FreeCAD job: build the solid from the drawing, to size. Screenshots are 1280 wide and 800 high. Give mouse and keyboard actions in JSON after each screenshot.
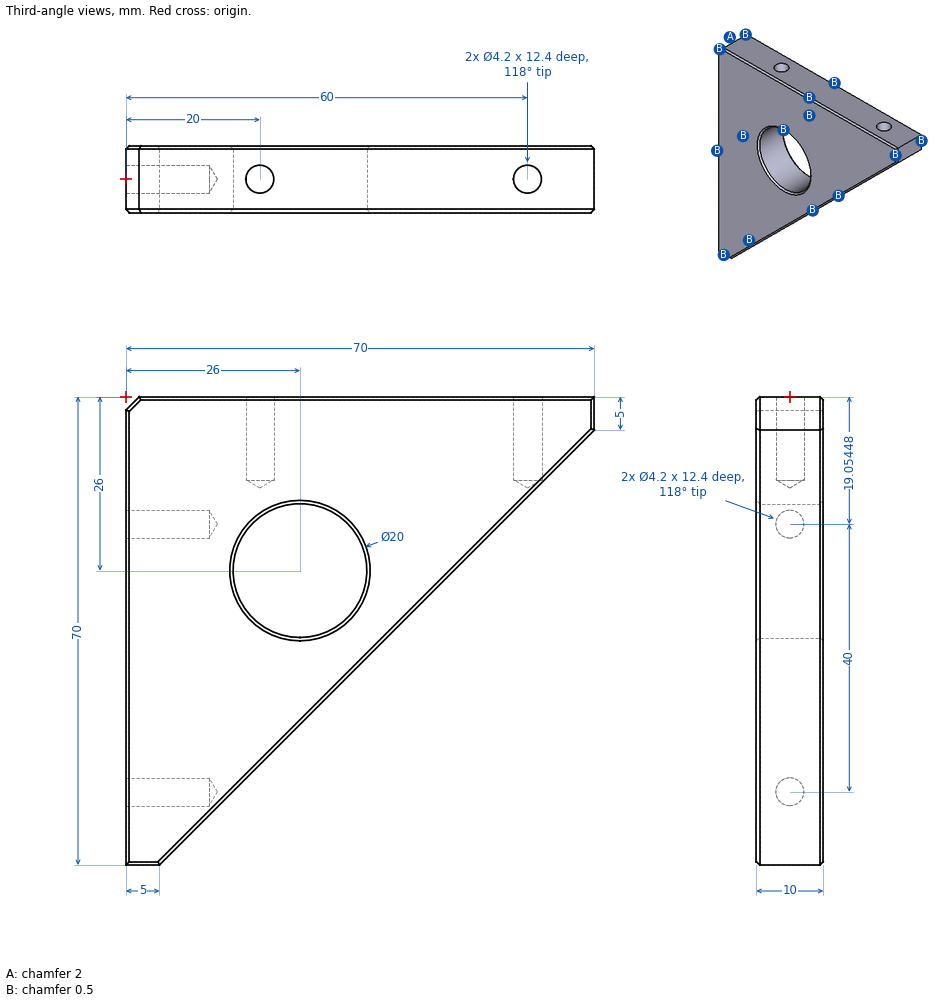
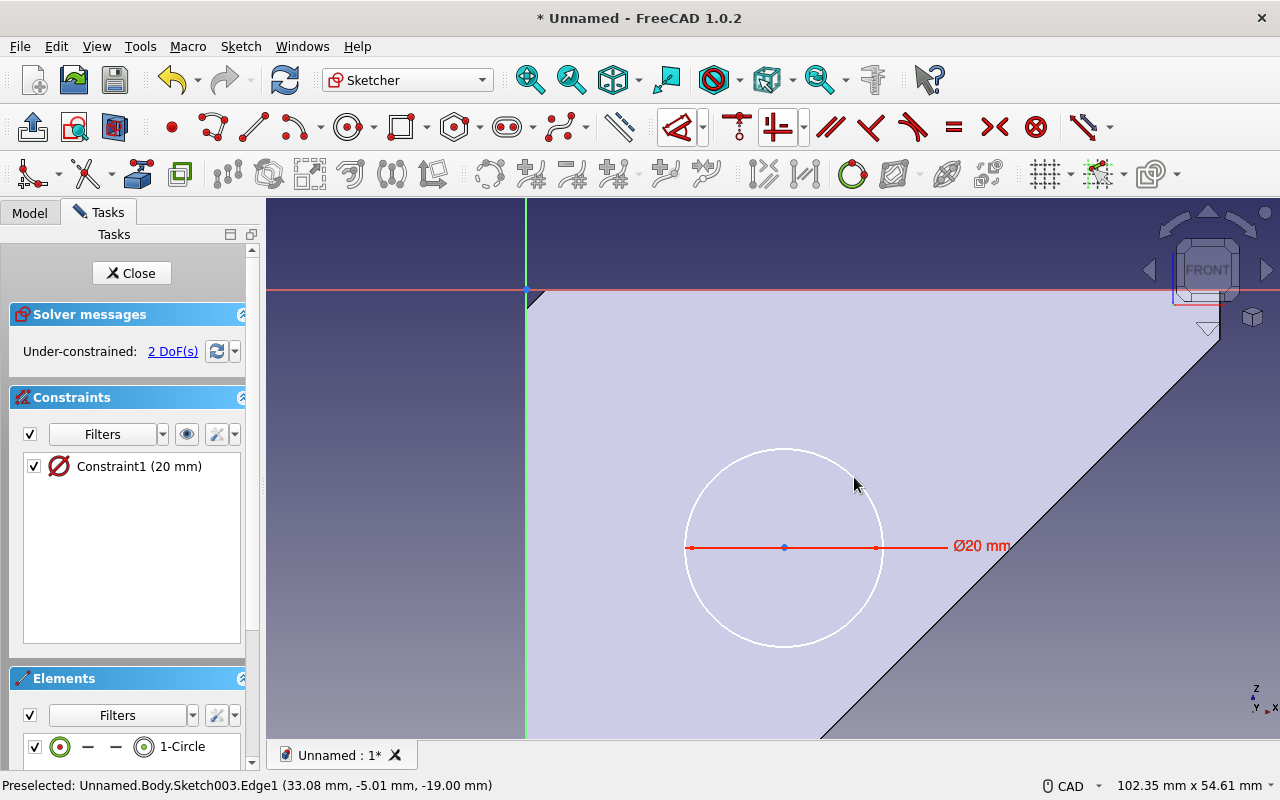
{"action": "left_click", "coordinate": [784, 548]}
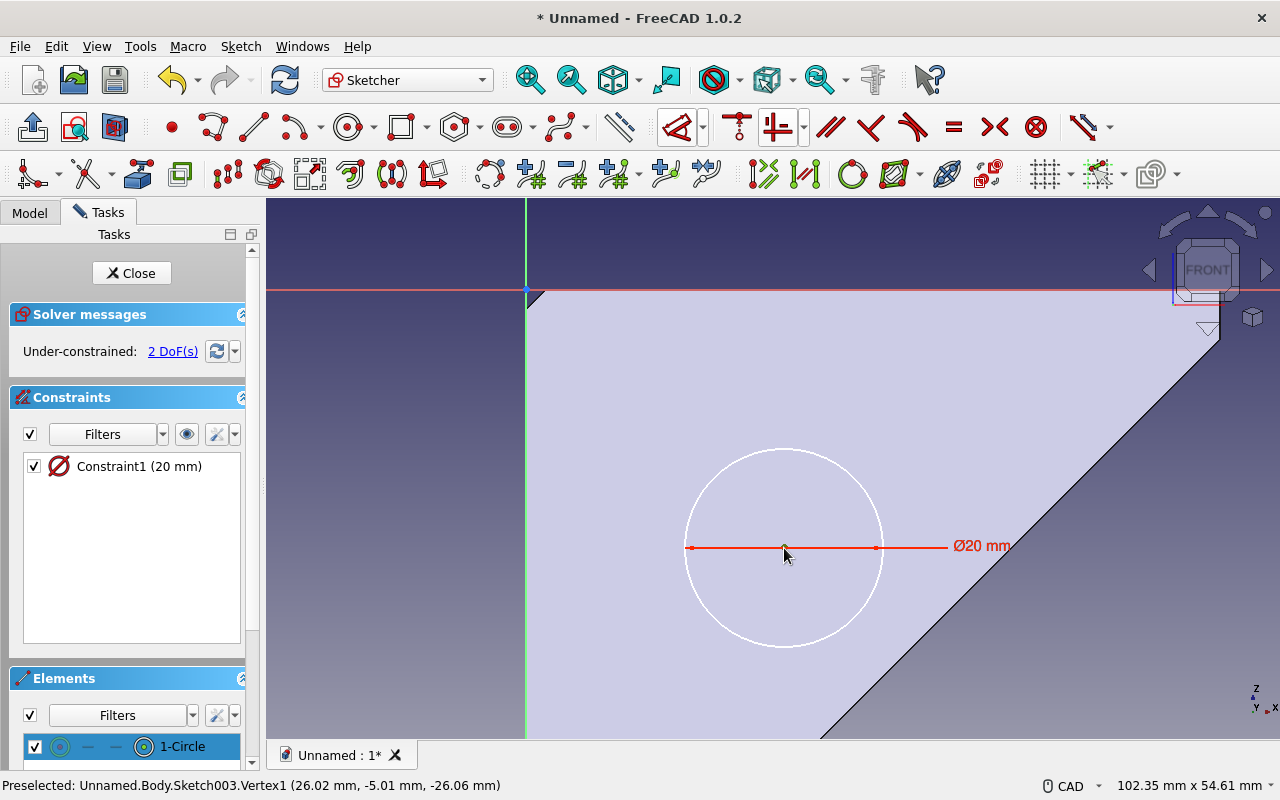
{"action": "key", "text": "l"}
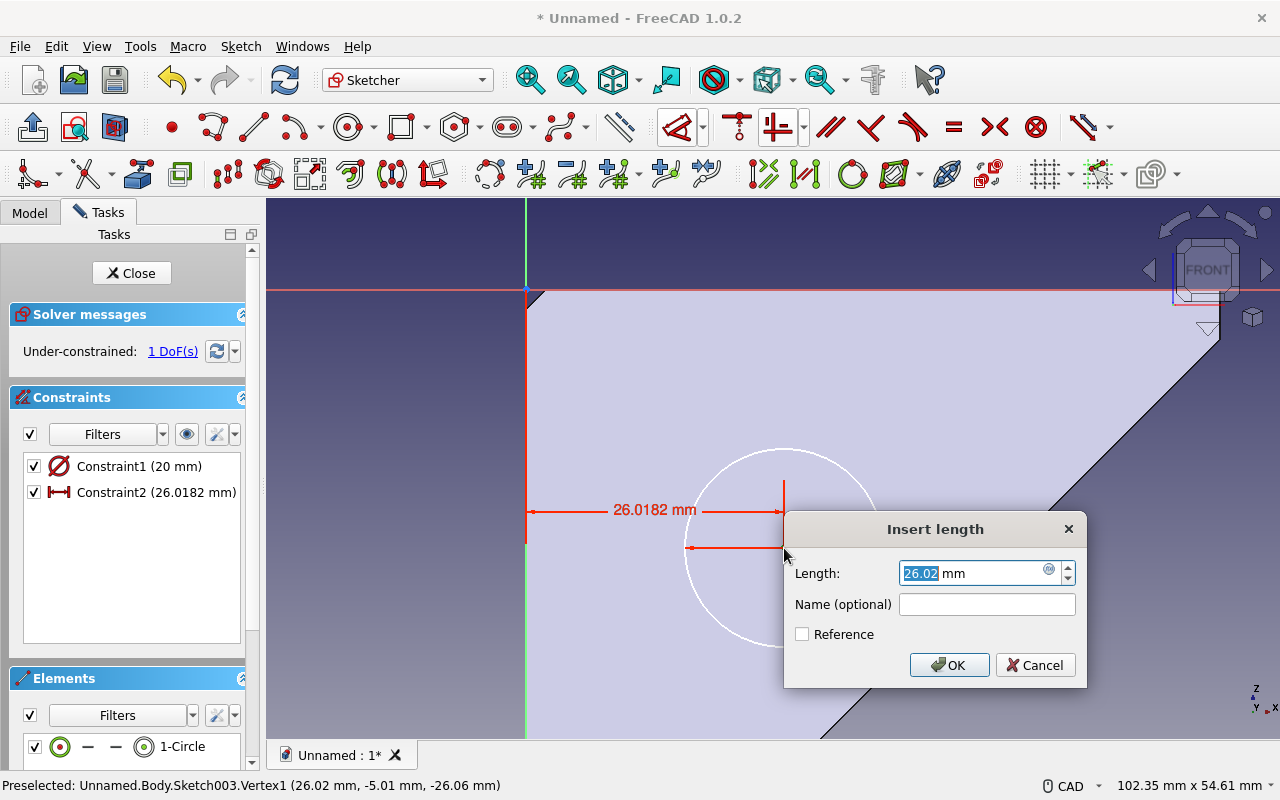
{"action": "type", "text": "26"}
{"action": "key", "text": "Return"}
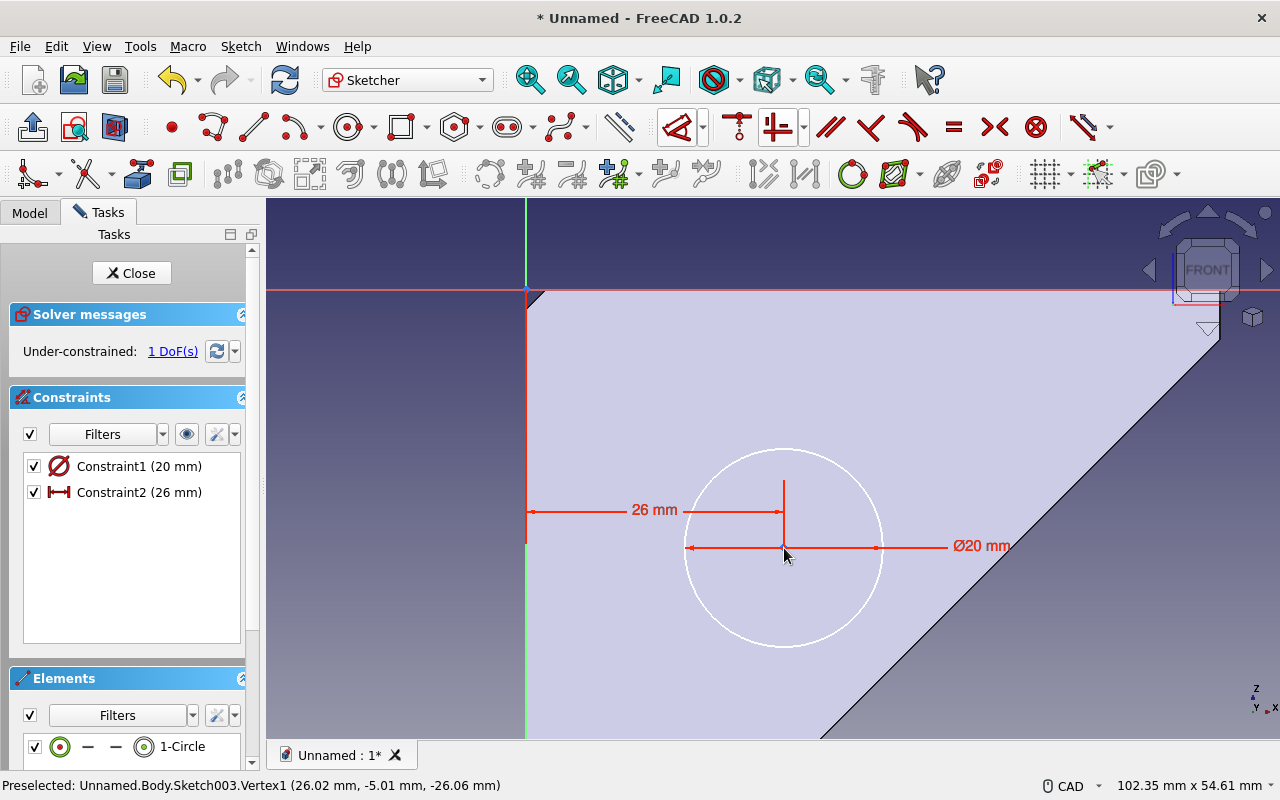
{"action": "left_click", "coordinate": [784, 548]}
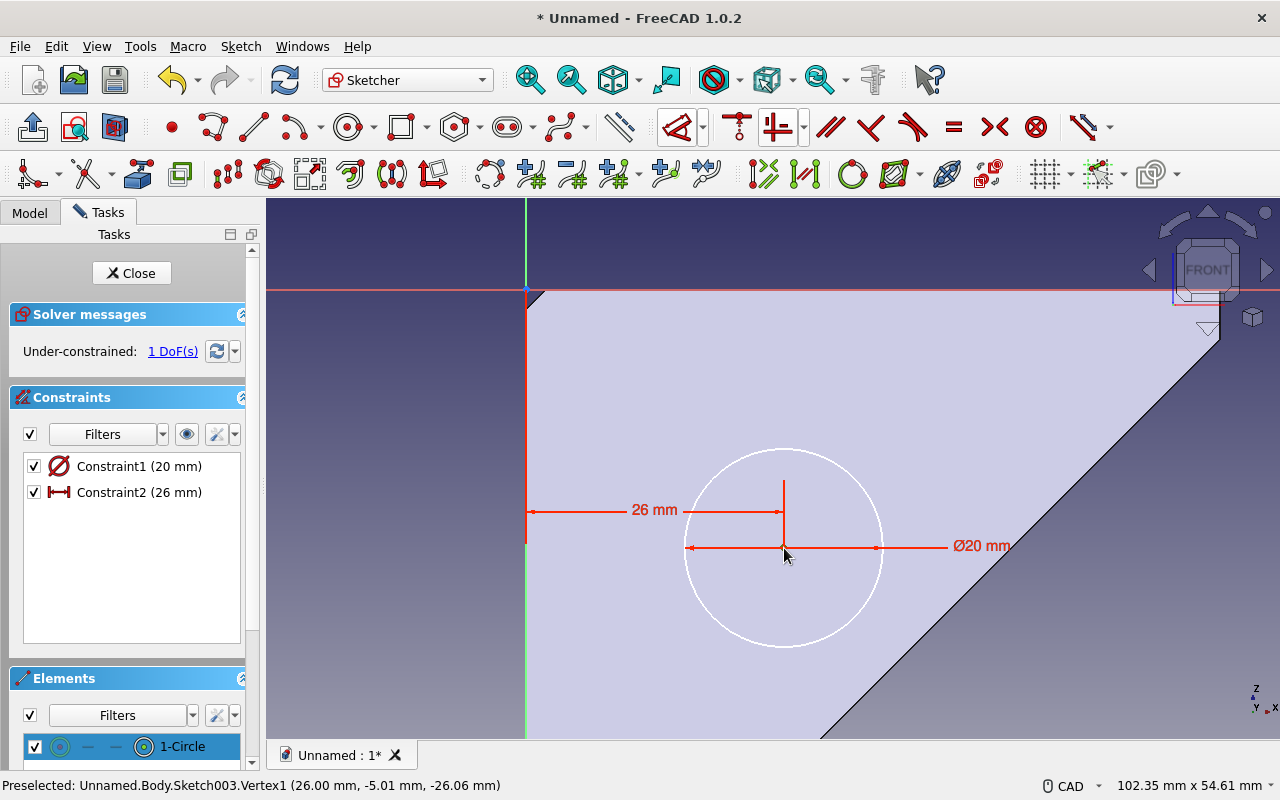
{"action": "left_click", "coordinate": [702, 128]}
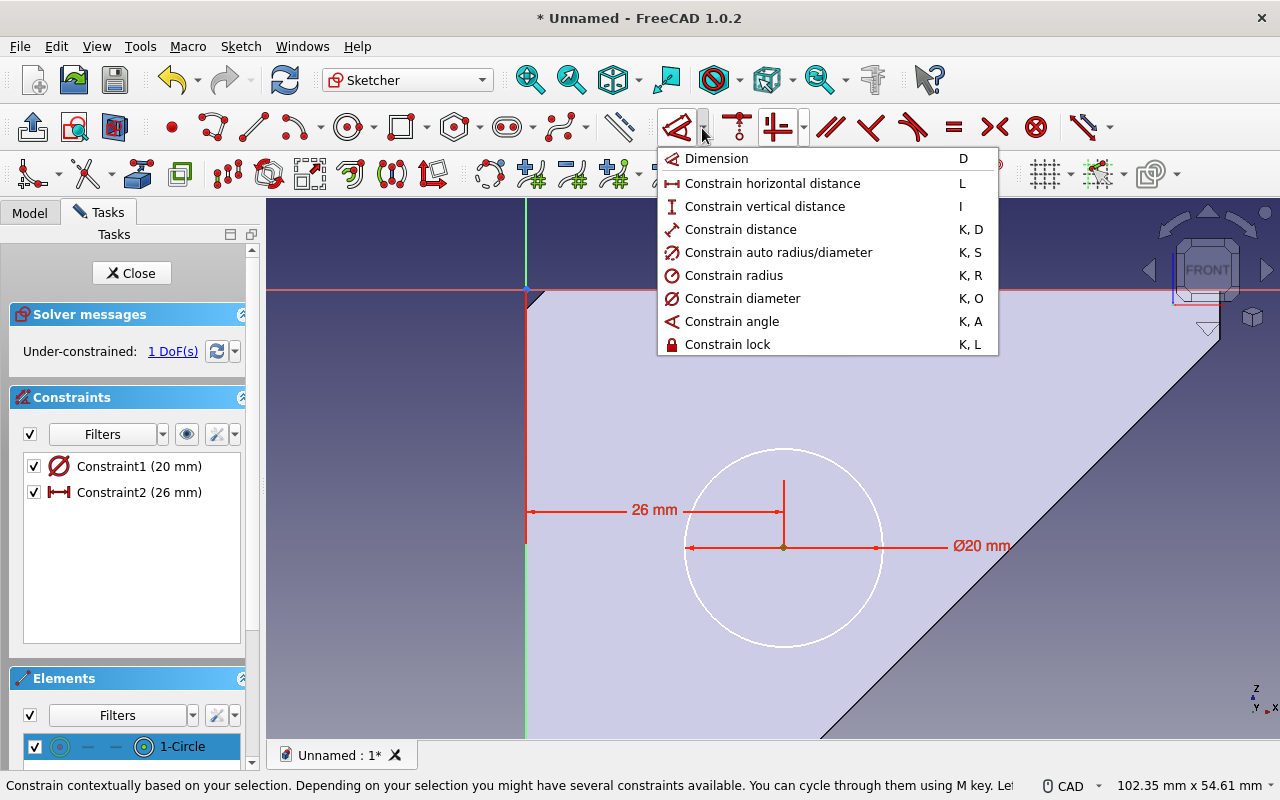
{"action": "left_click", "coordinate": [828, 206]}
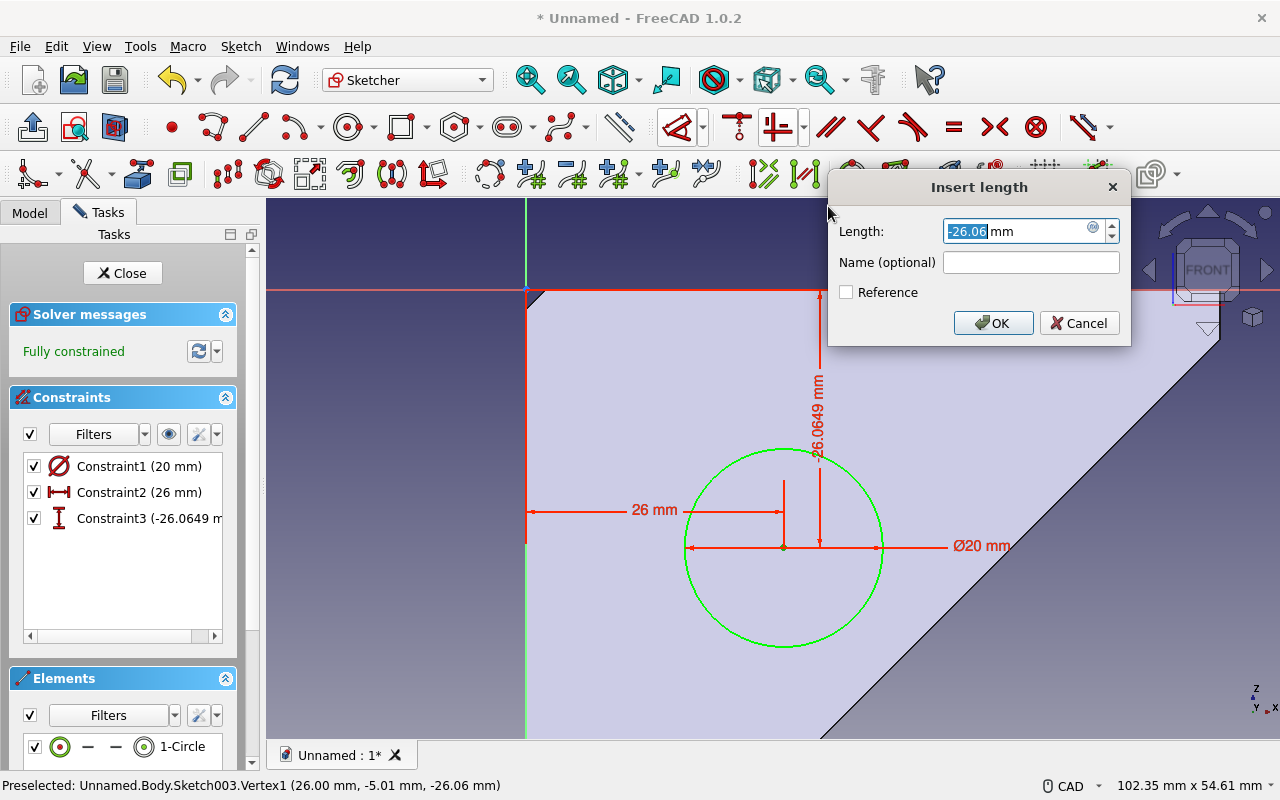
{"action": "type", "text": "-26"}
{"action": "key", "text": "Return"}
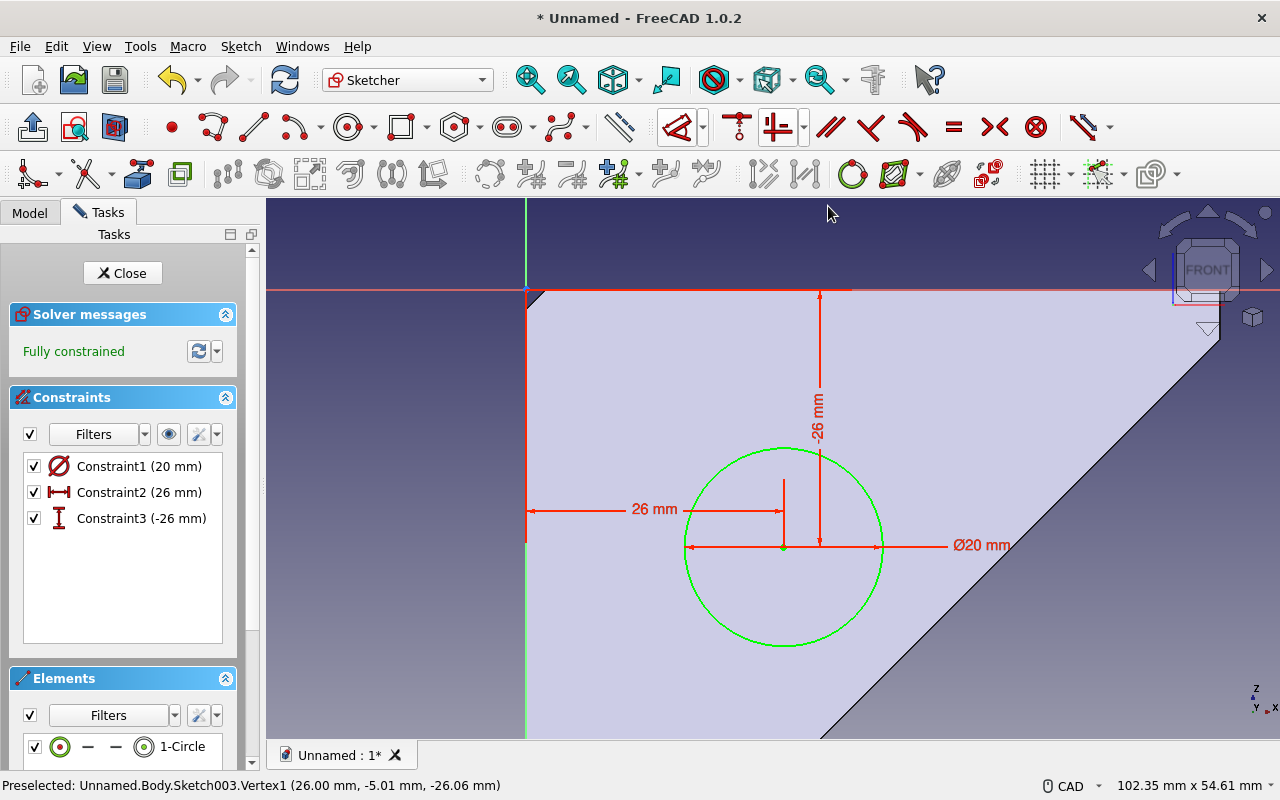
{"action": "left_click", "coordinate": [123, 273]}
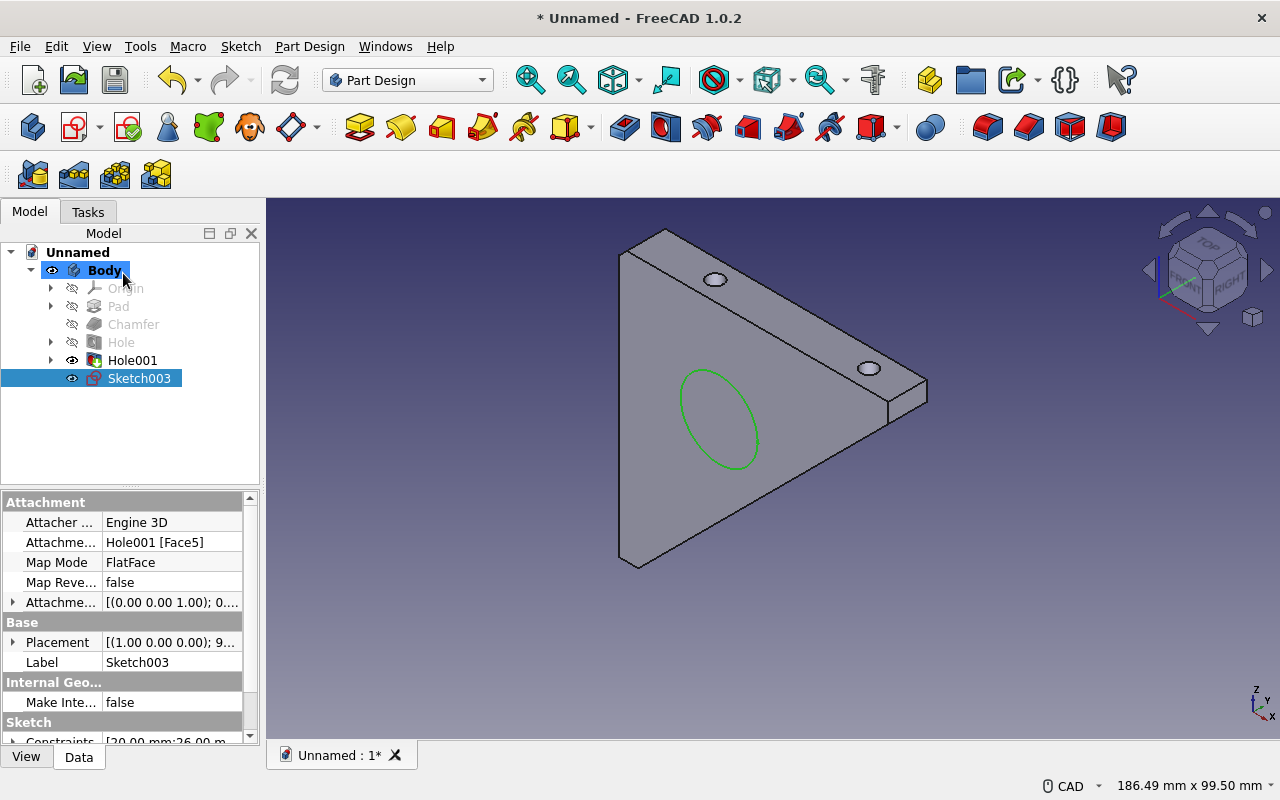
{"action": "left_click", "coordinate": [625, 128]}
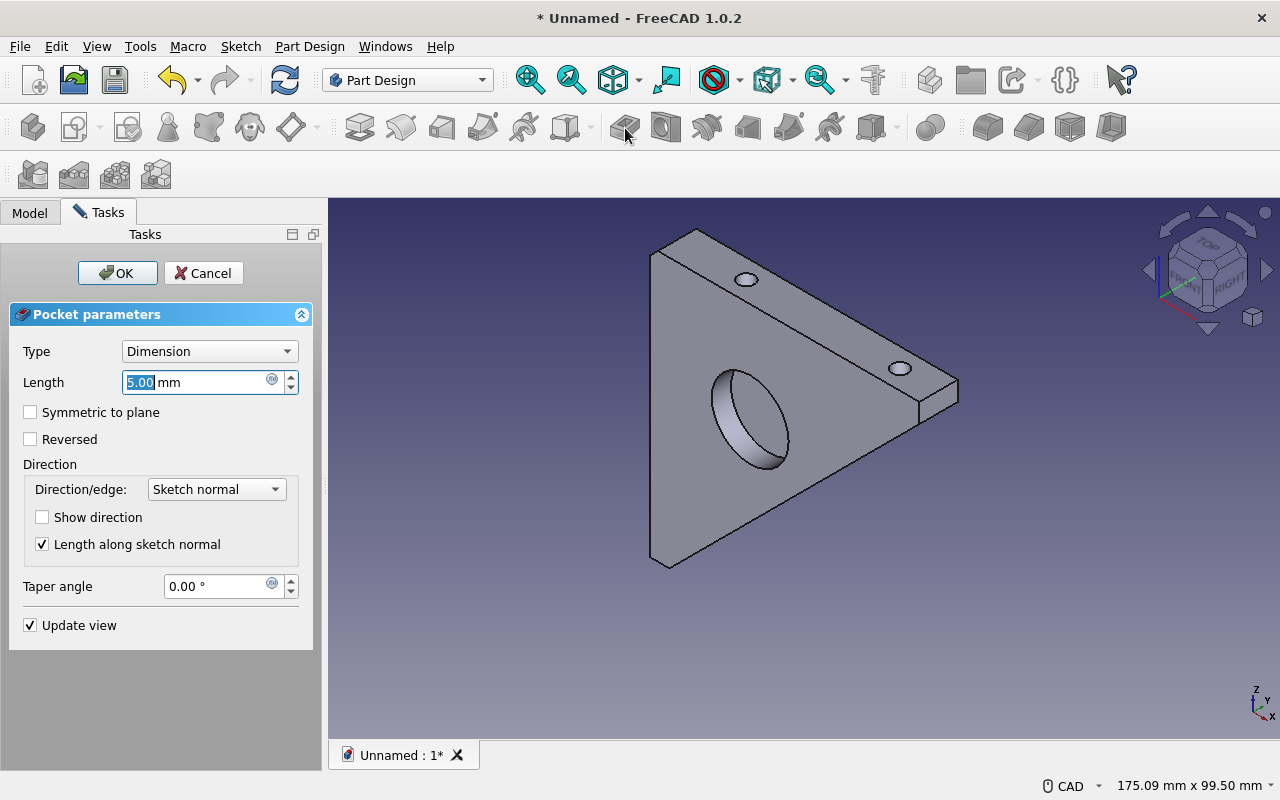
{"action": "left_click", "coordinate": [210, 352]}